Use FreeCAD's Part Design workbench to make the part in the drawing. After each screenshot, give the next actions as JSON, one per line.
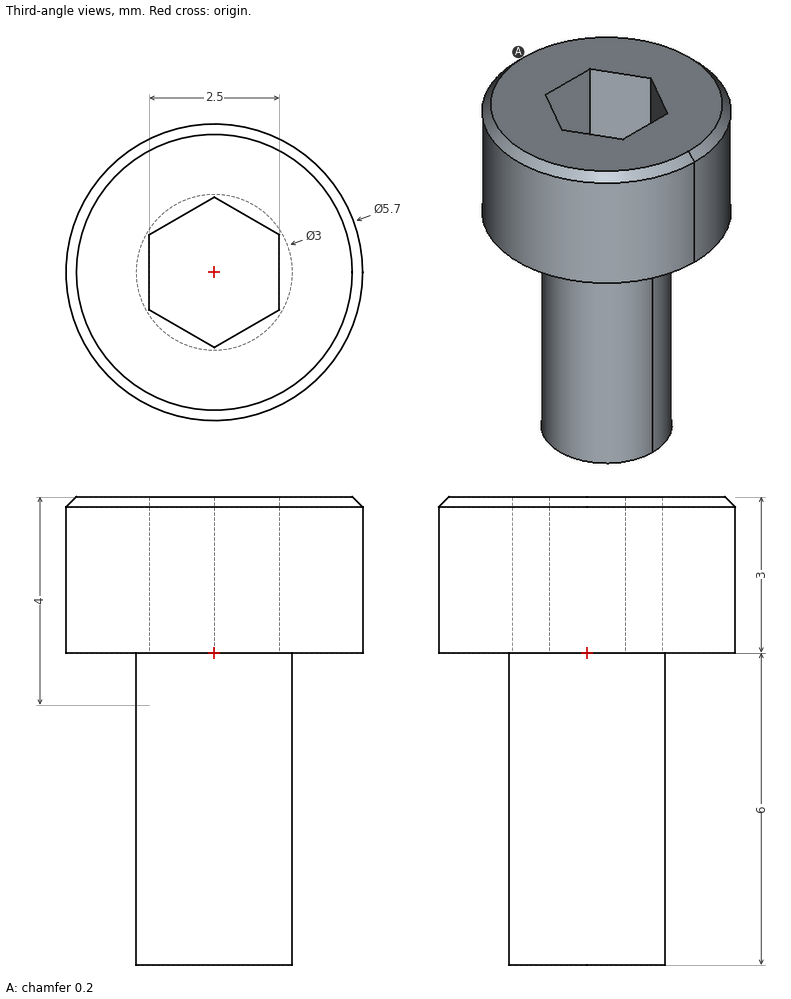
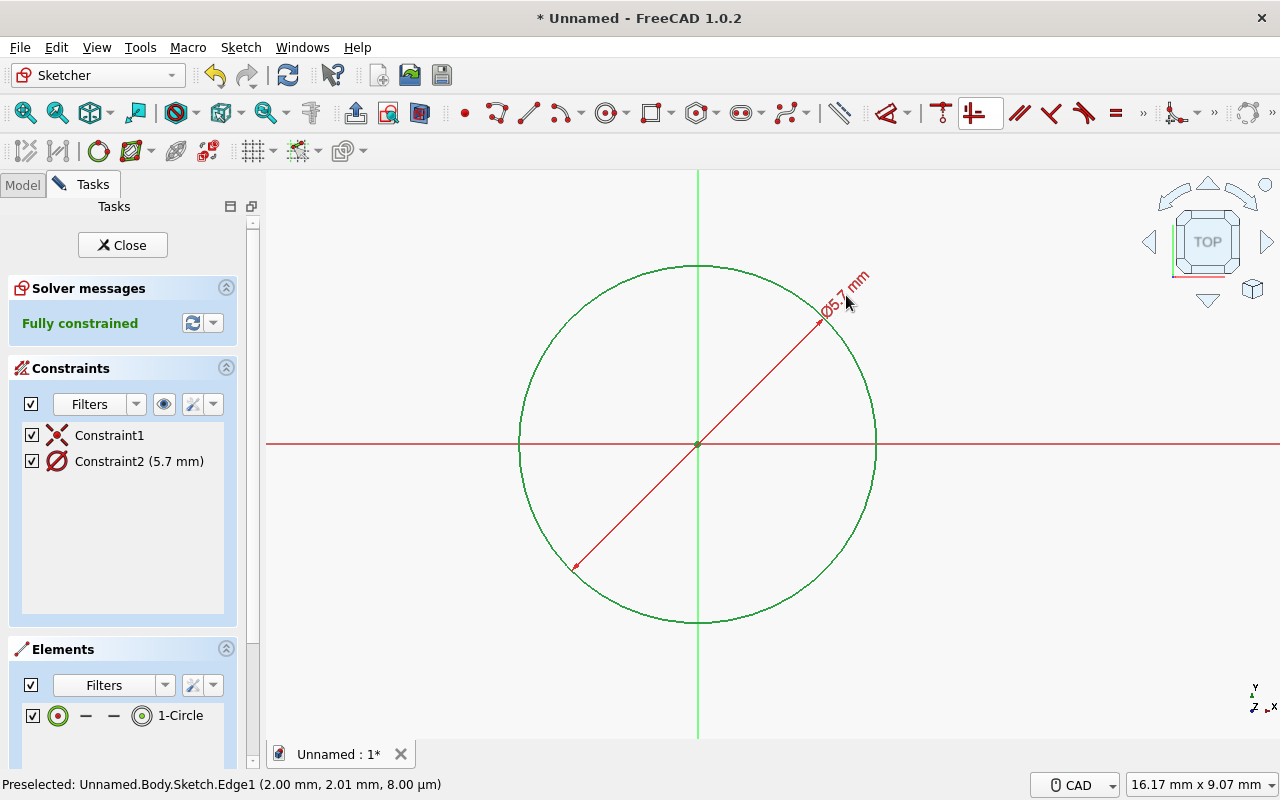
{"action": "left_click", "coordinate": [123, 245]}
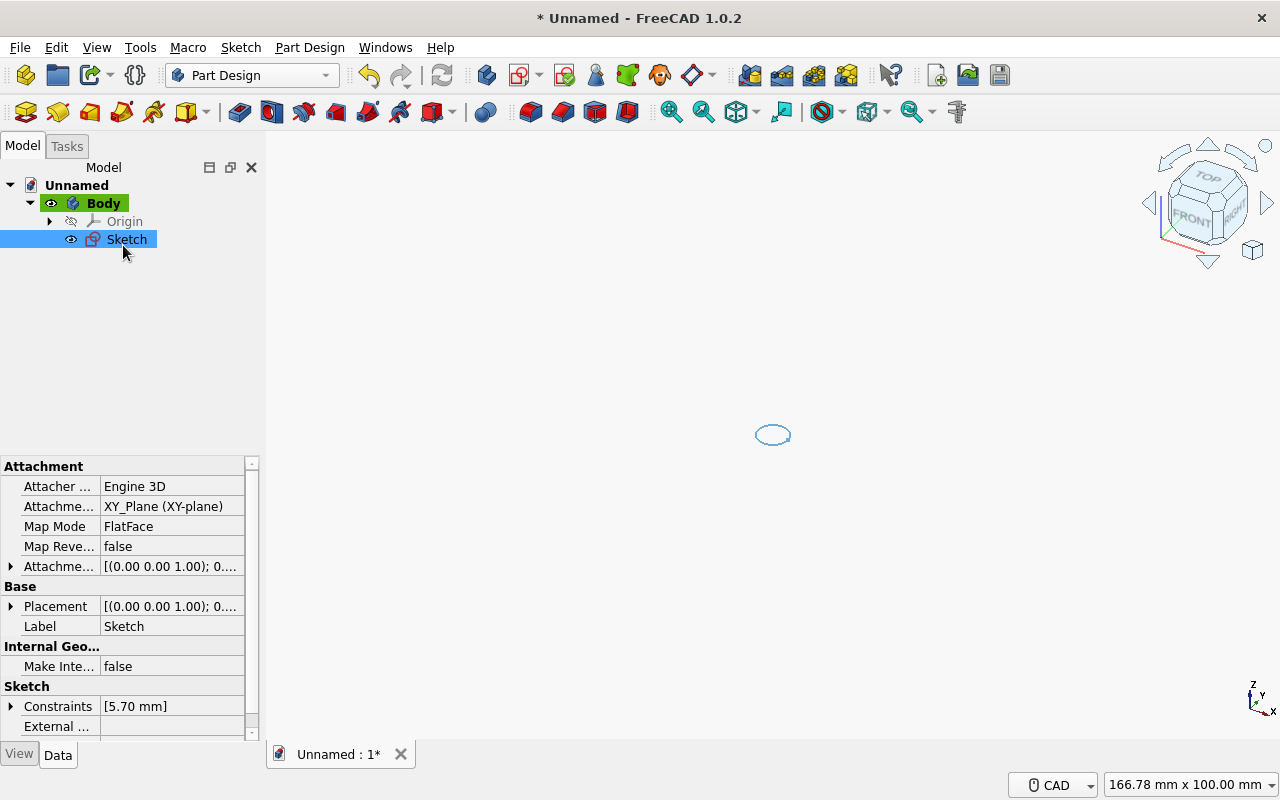
{"action": "left_click", "coordinate": [26, 112]}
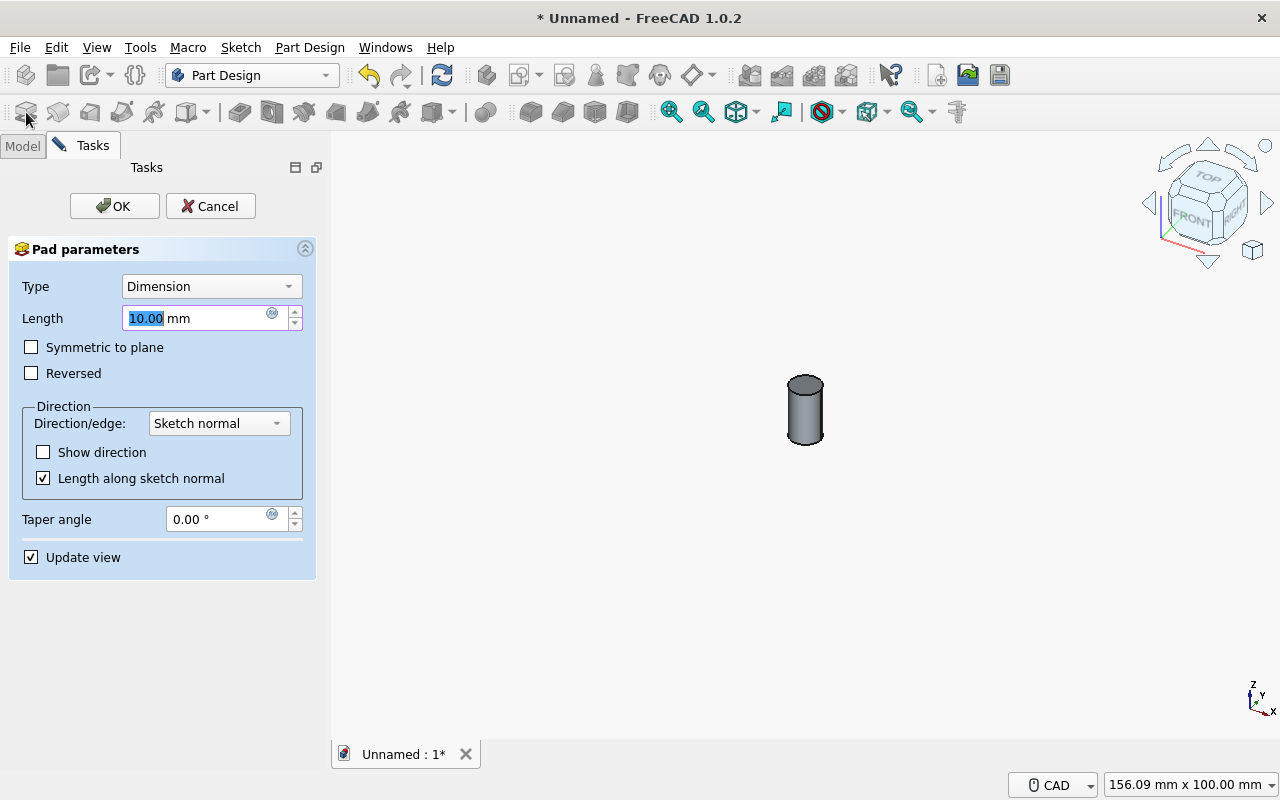
{"action": "type", "text": "3"}
{"action": "key", "text": "Tab"}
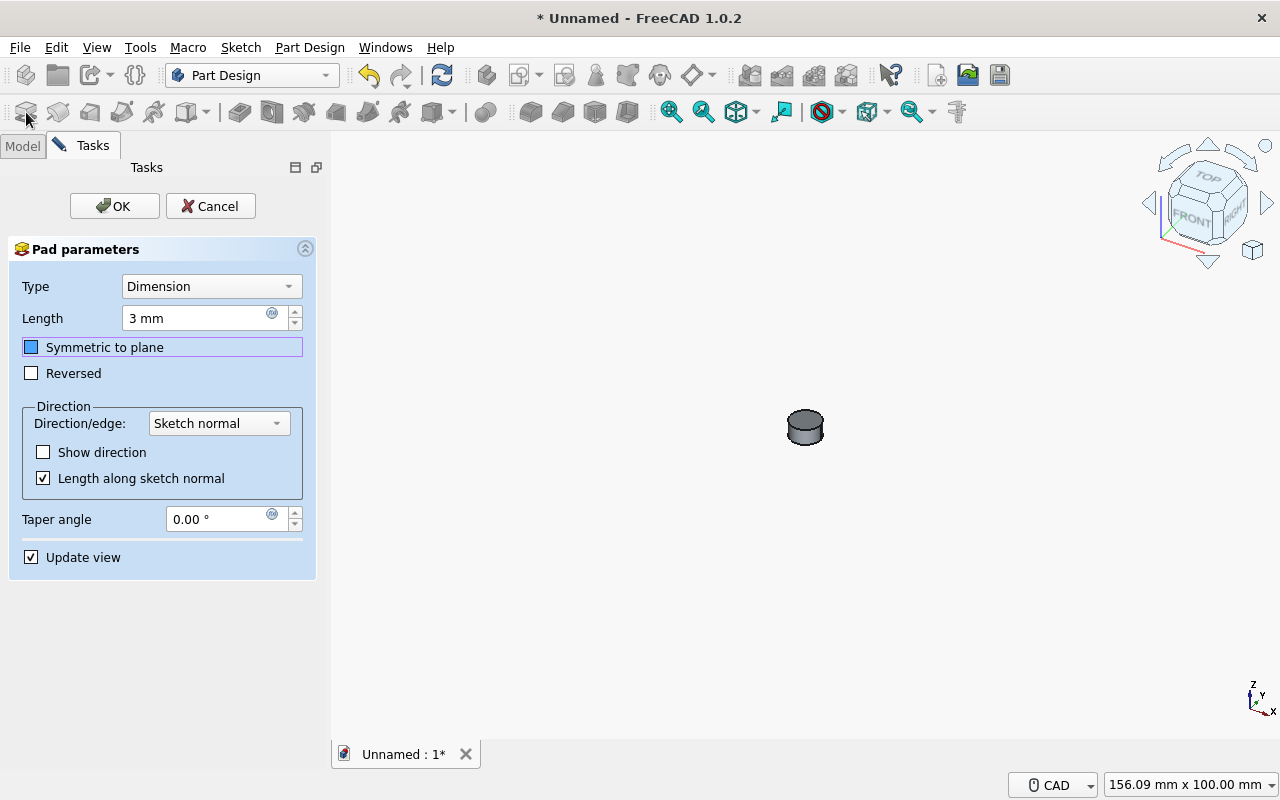
{"action": "left_click", "coordinate": [115, 206]}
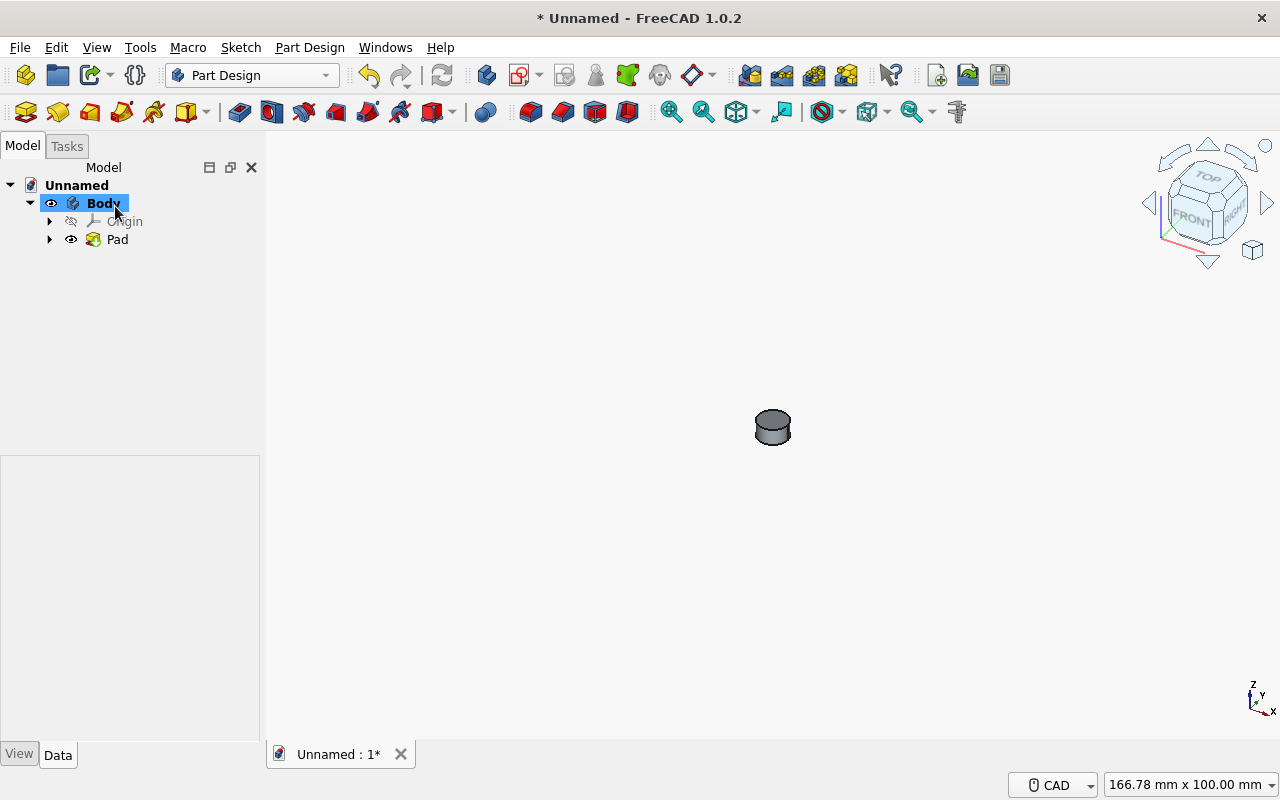
{"action": "left_click", "coordinate": [672, 112]}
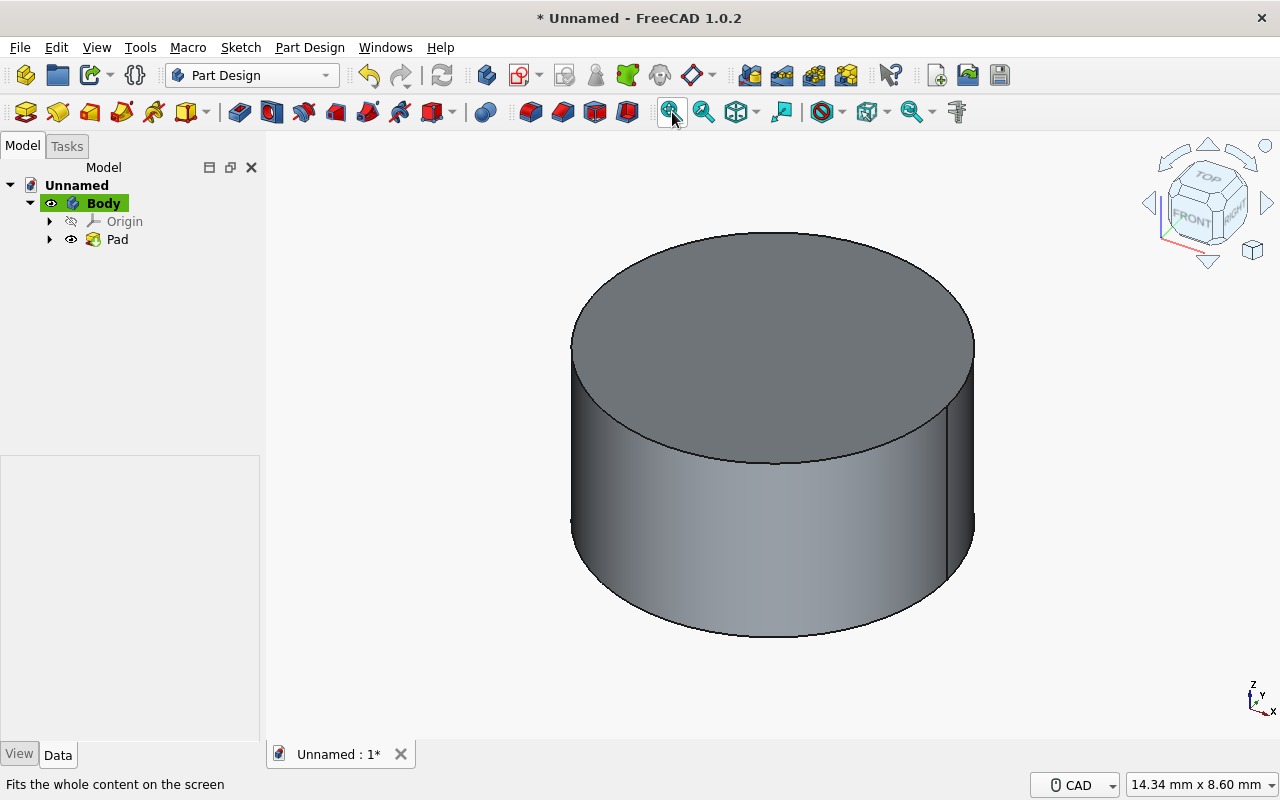
{"action": "left_click", "coordinate": [773, 347]}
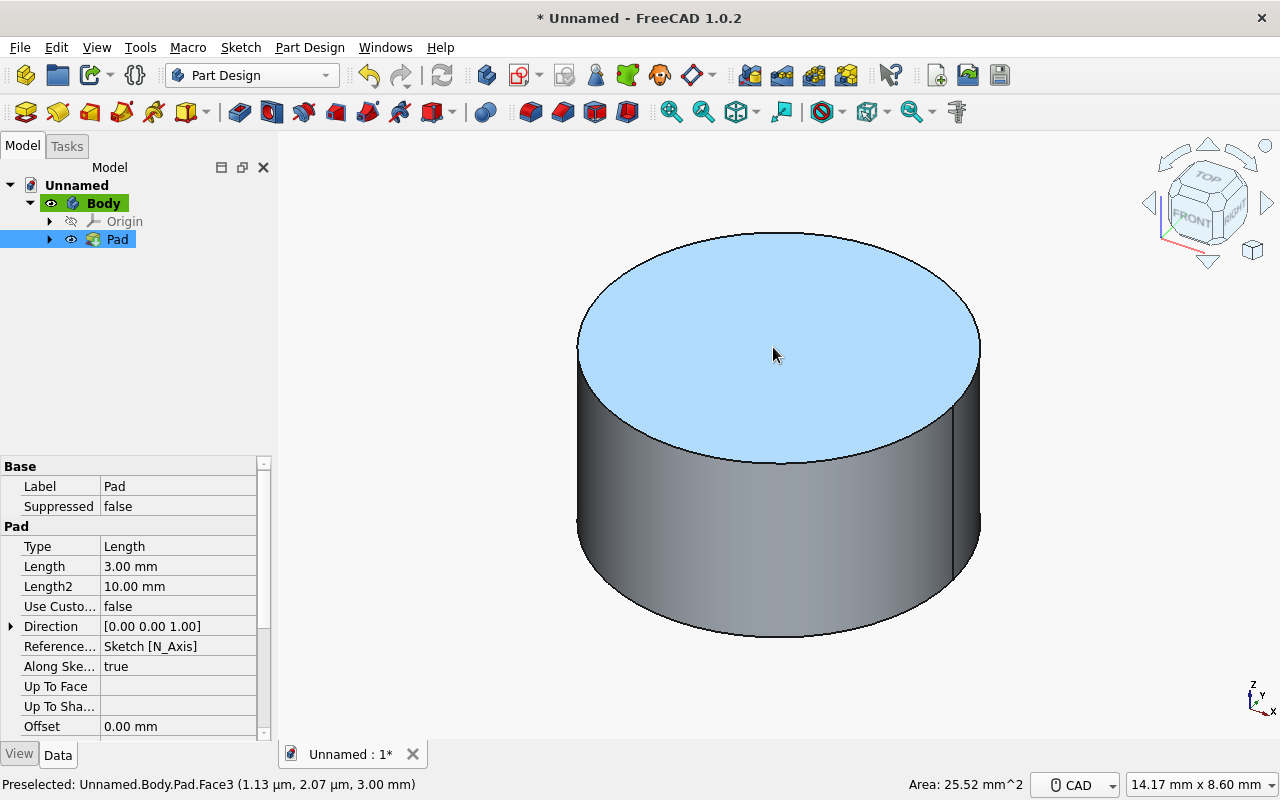
{"action": "left_click", "coordinate": [520, 76]}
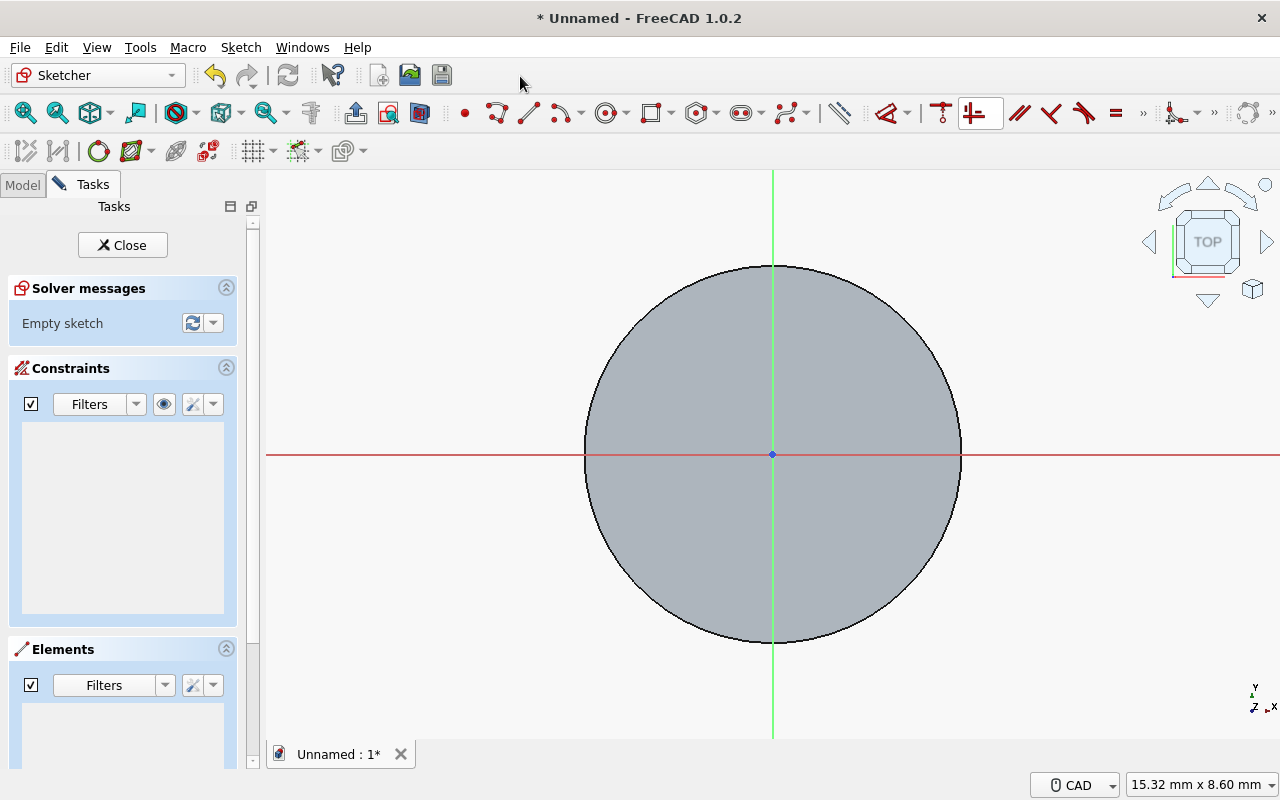
{"action": "scroll", "coordinate": [856, 454], "scroll_direction": "up", "scroll_amount": 3}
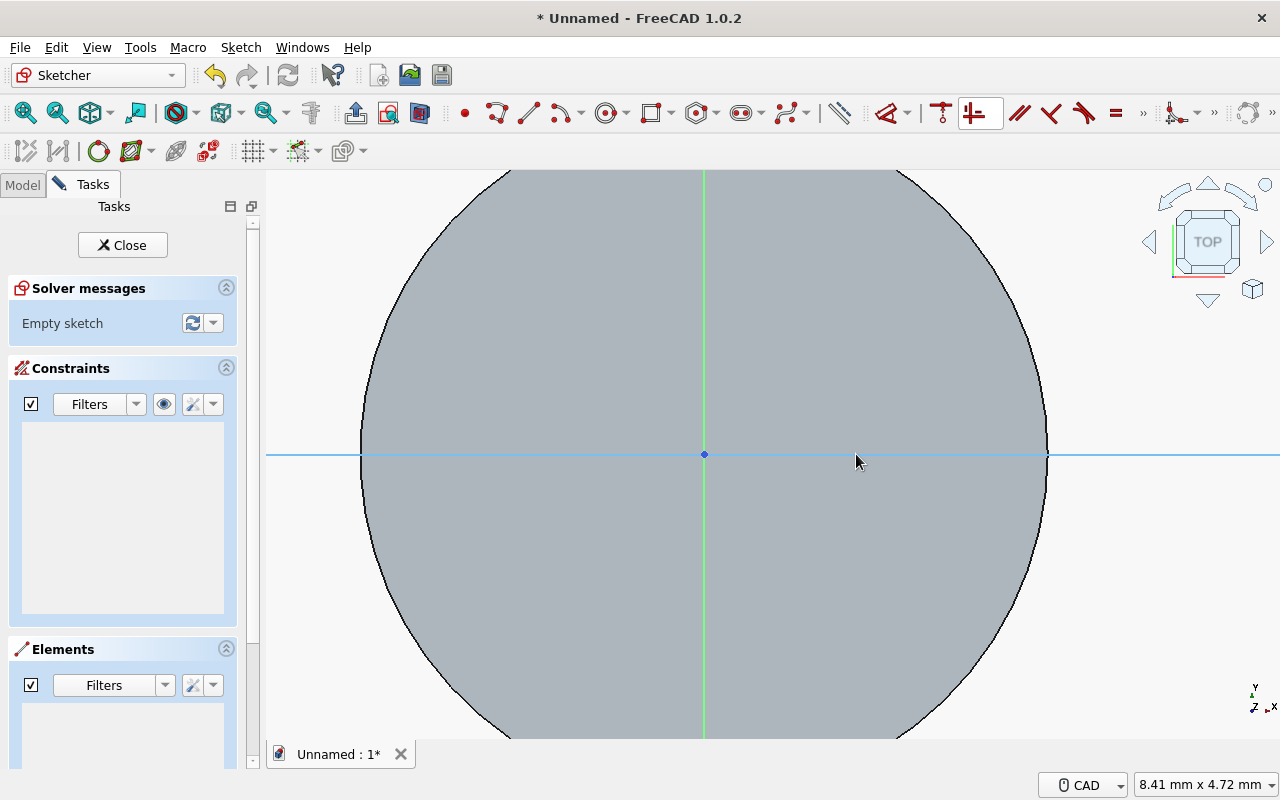
{"action": "left_click", "coordinate": [696, 114]}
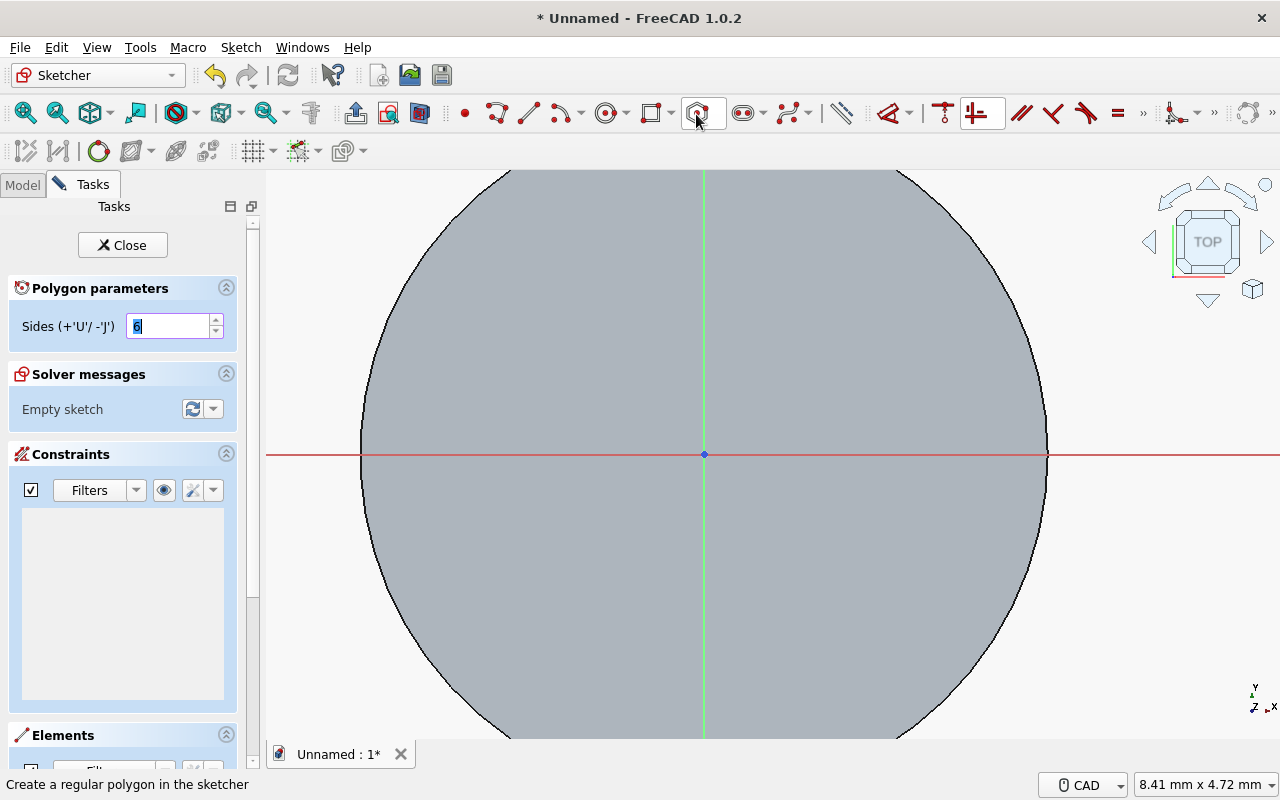
{"action": "left_click", "coordinate": [704, 454]}